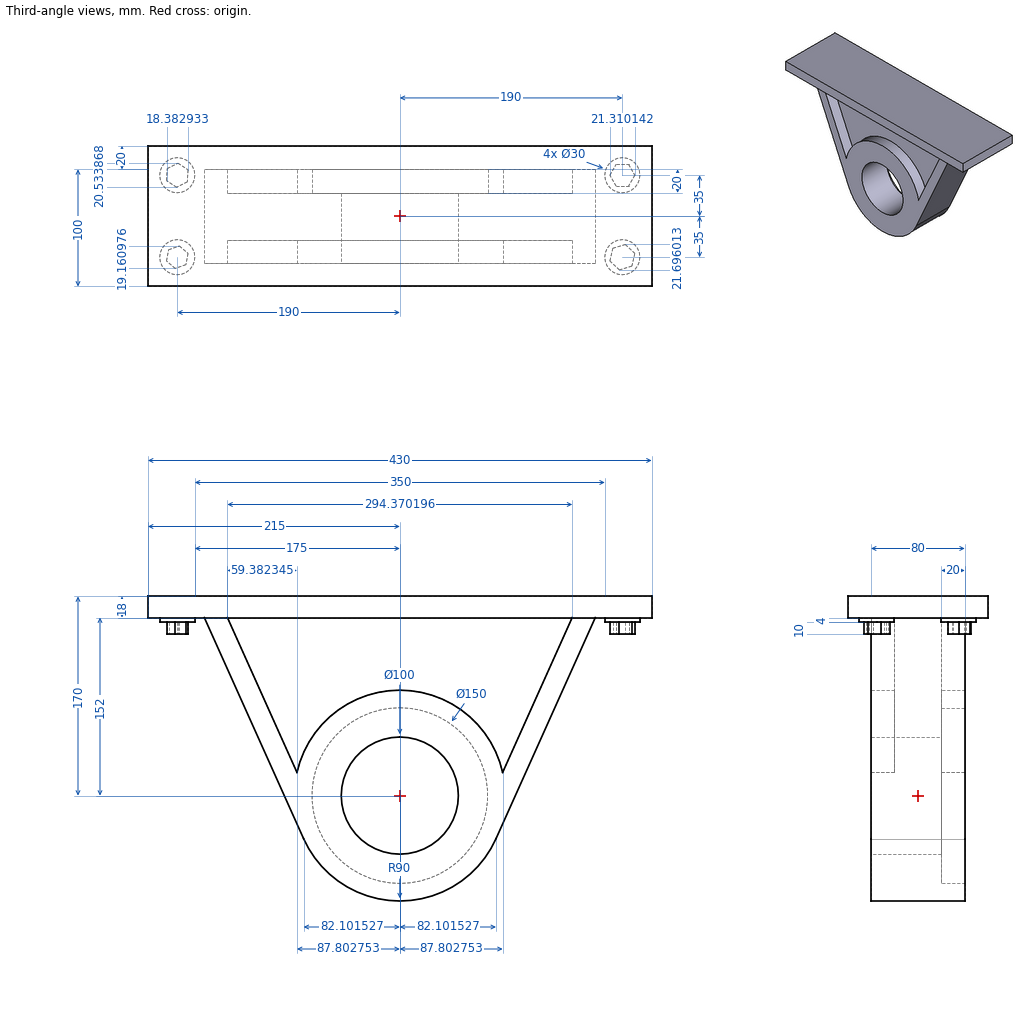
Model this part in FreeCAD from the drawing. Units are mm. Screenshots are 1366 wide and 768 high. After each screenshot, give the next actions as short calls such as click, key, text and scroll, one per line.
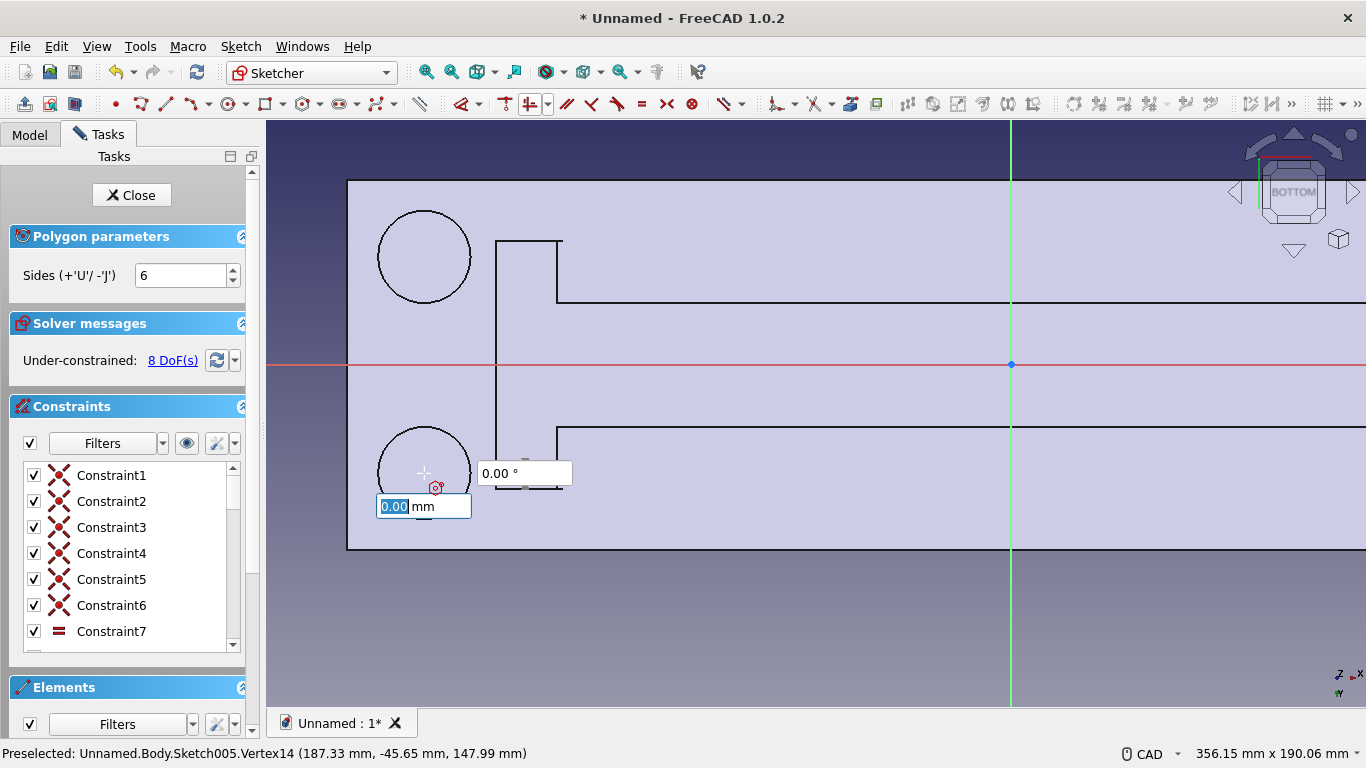
click(426, 505)
right_click(426, 505)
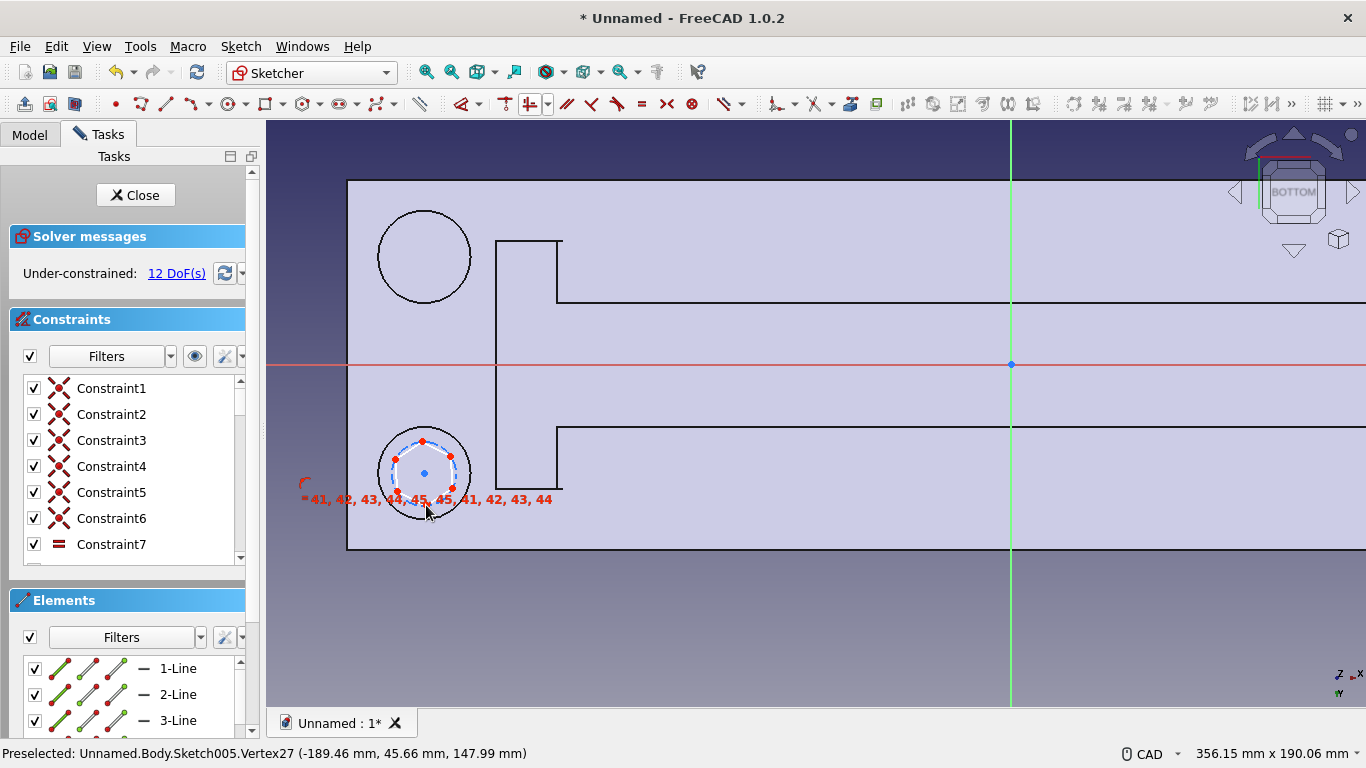
click(302, 104)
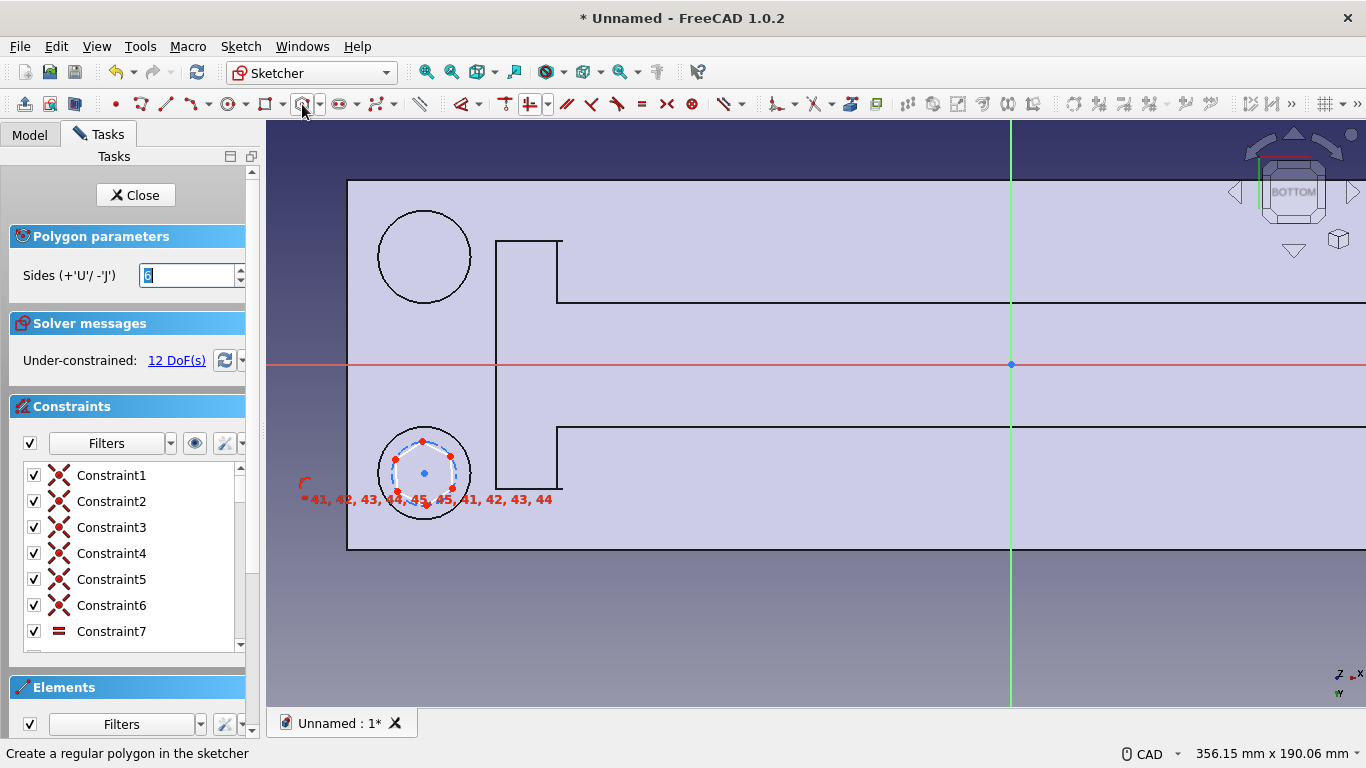
click(424, 257)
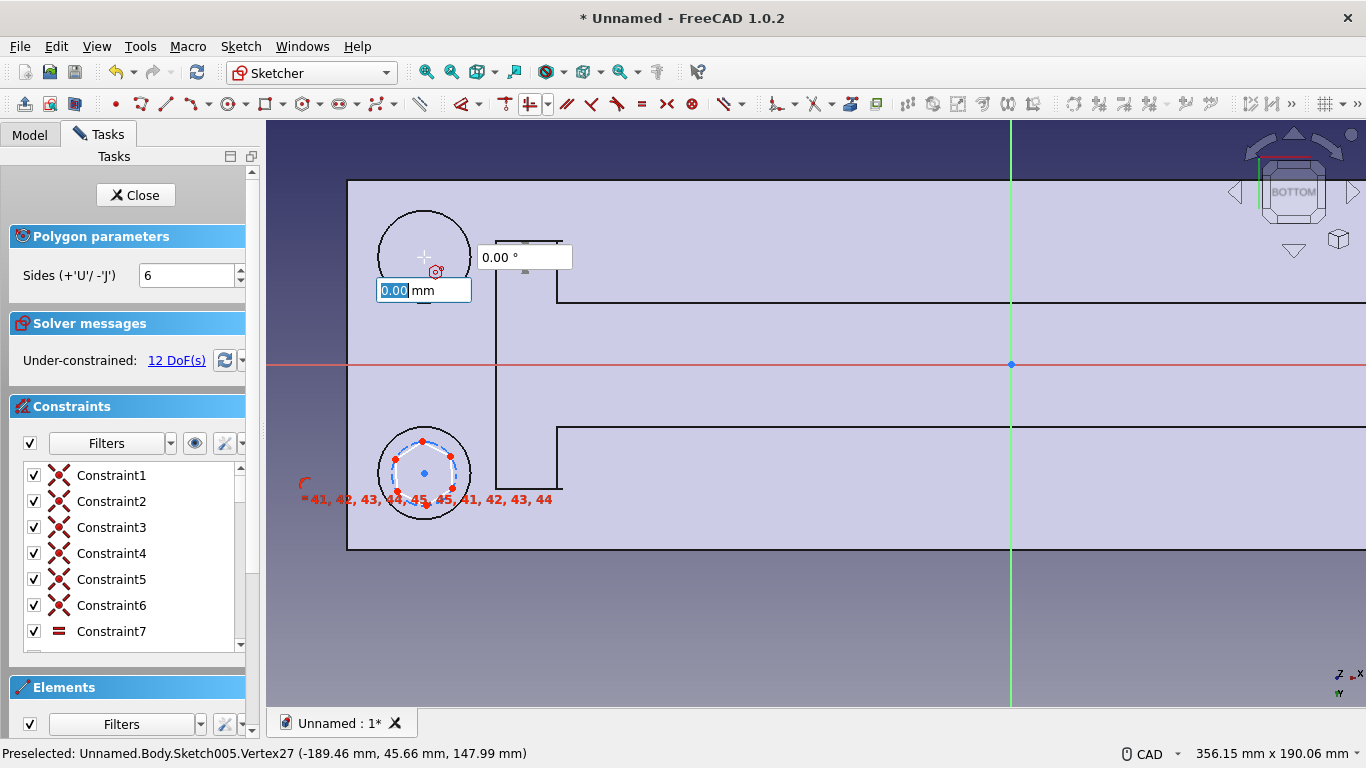
click(419, 227)
right_click(419, 227)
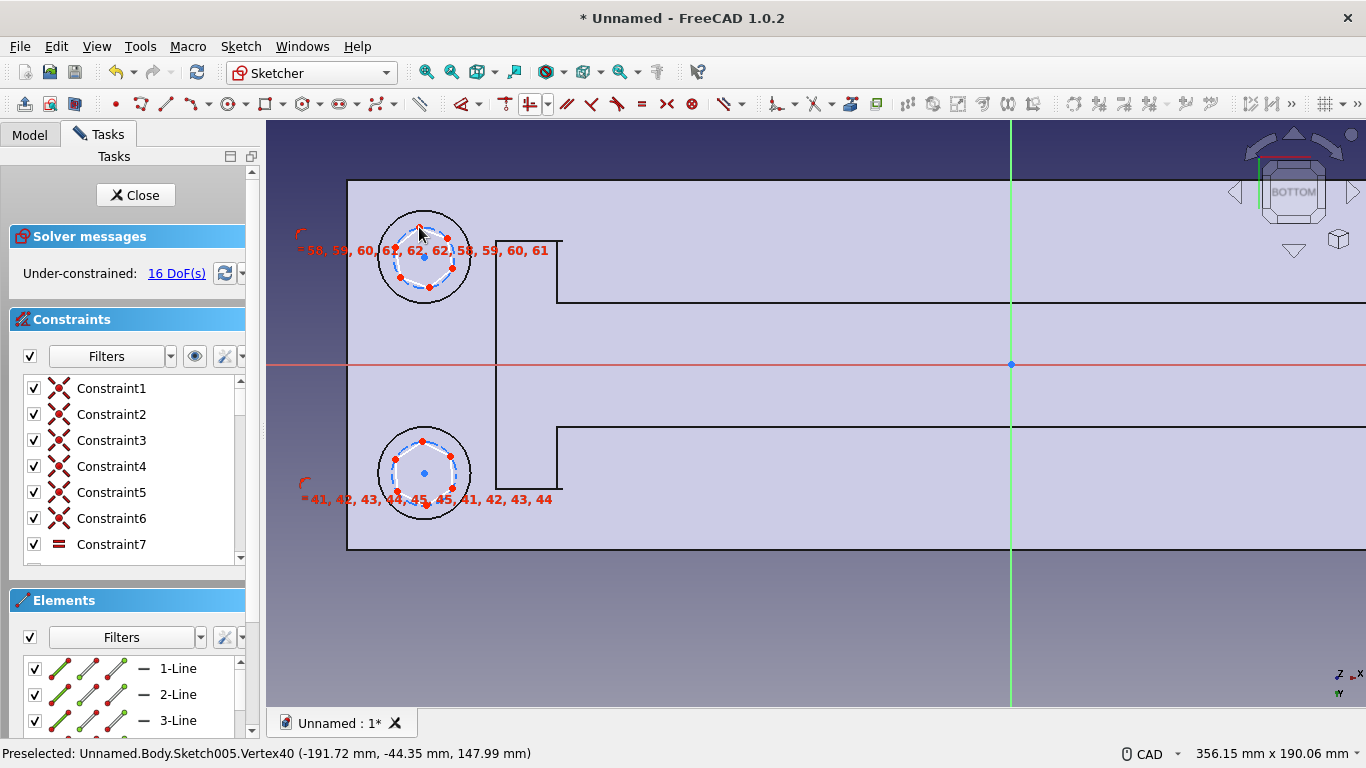
scroll(424, 474, down, 3)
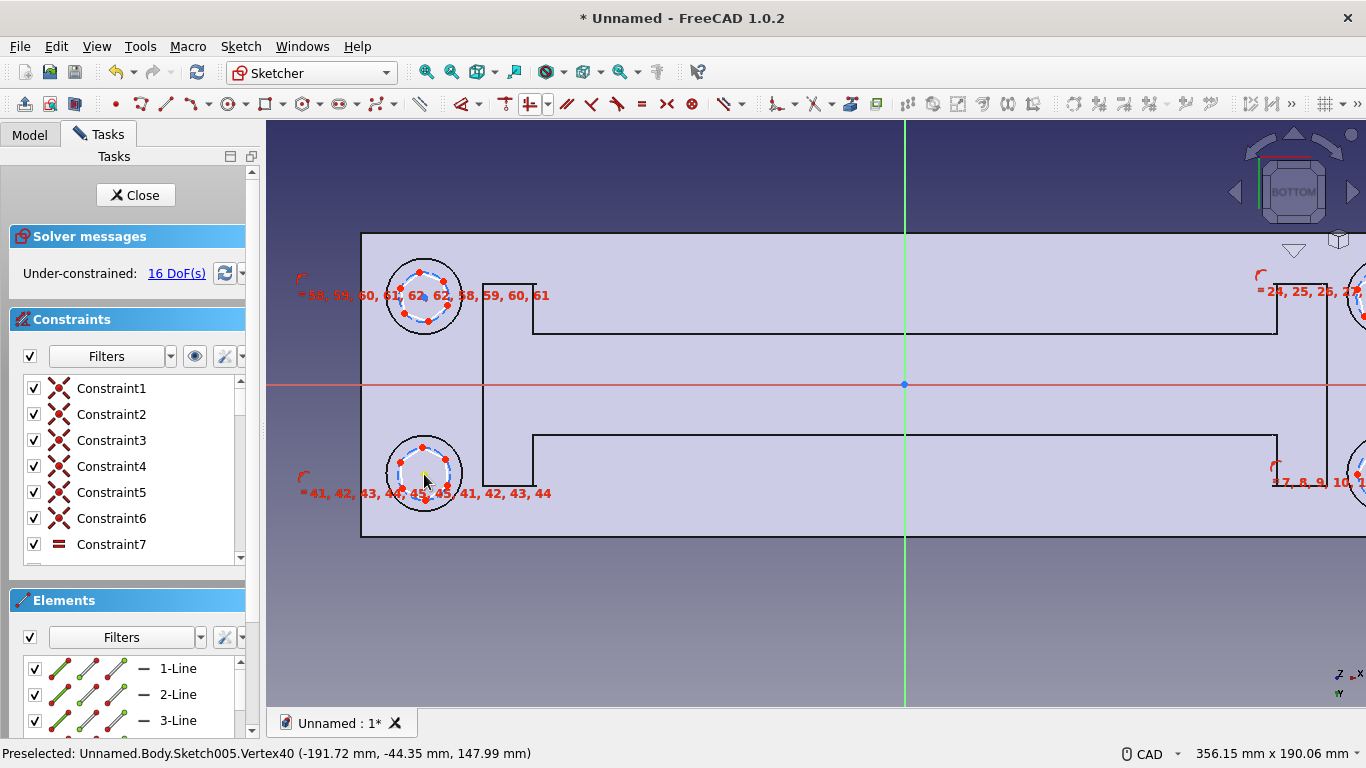
scroll(1068, 490, up, 9)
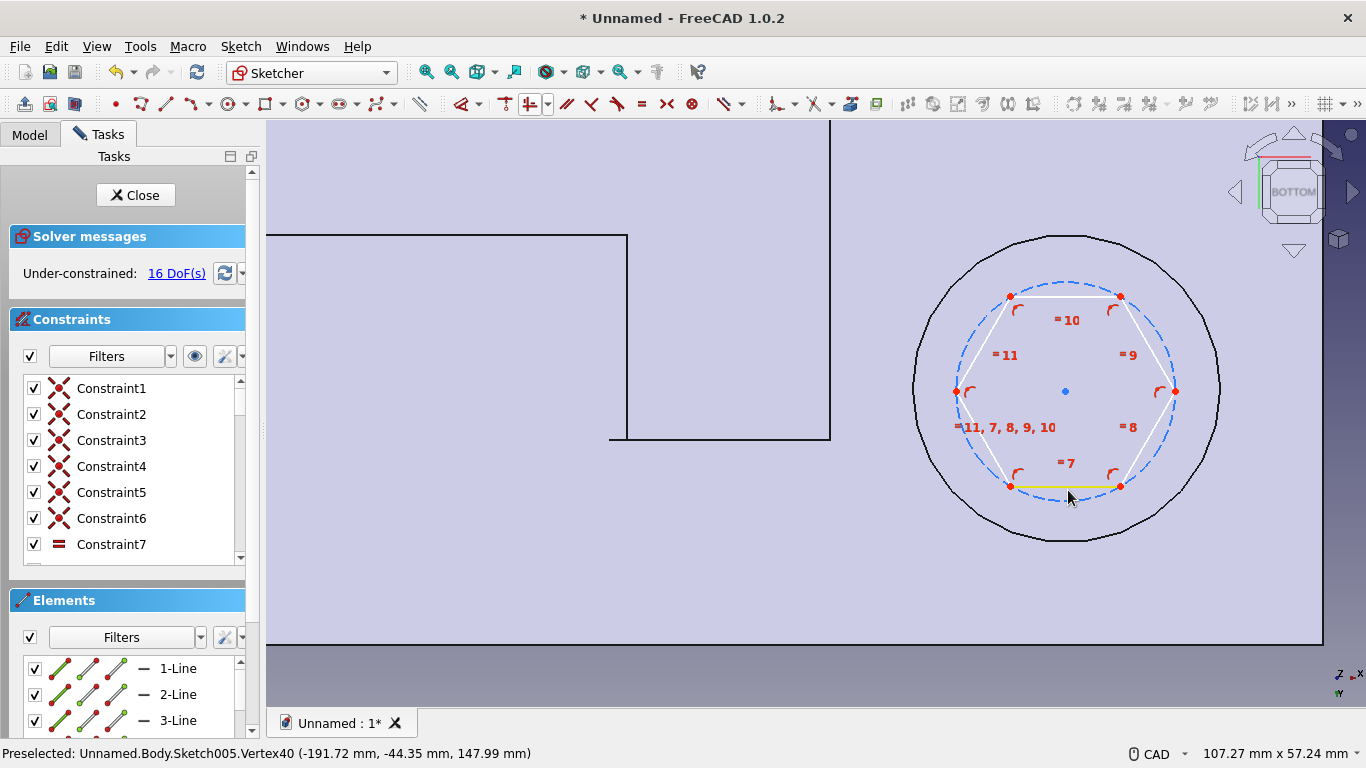
click(1066, 487)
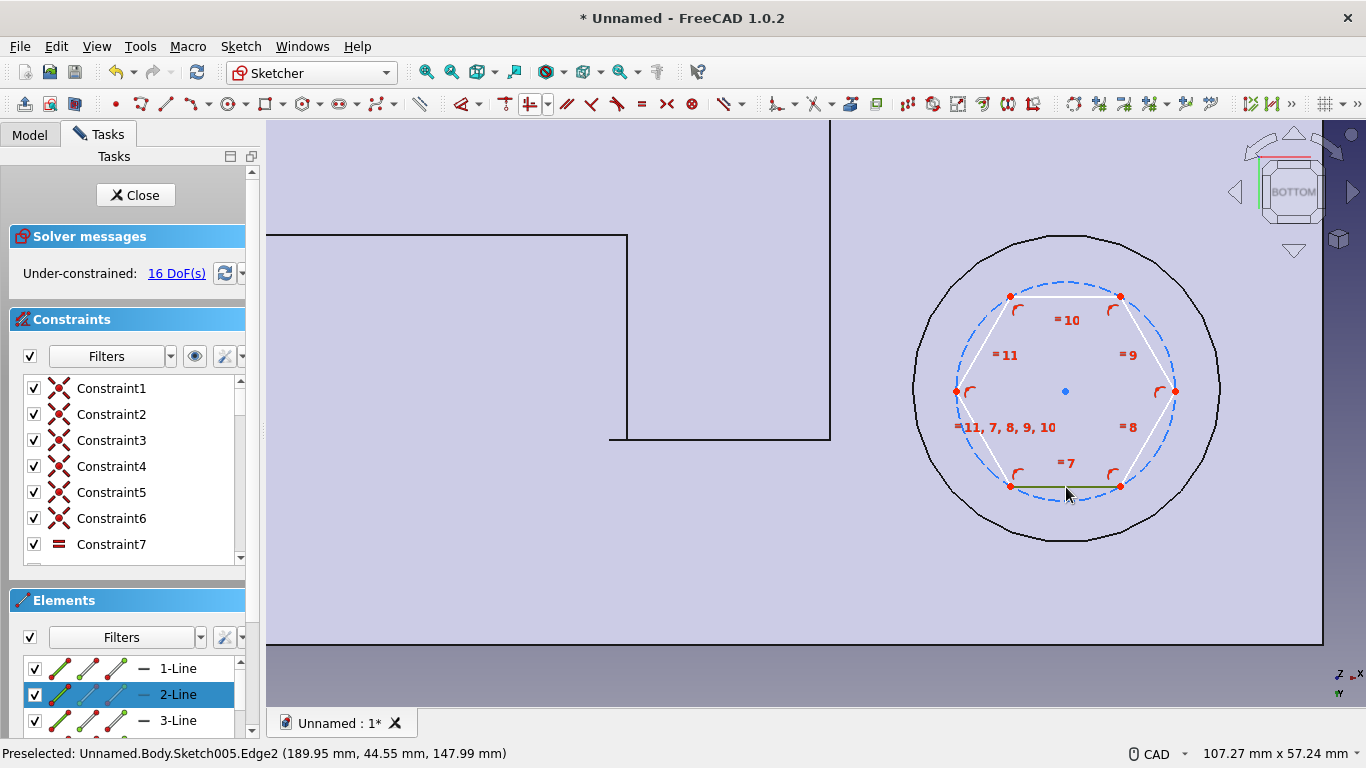
key(h)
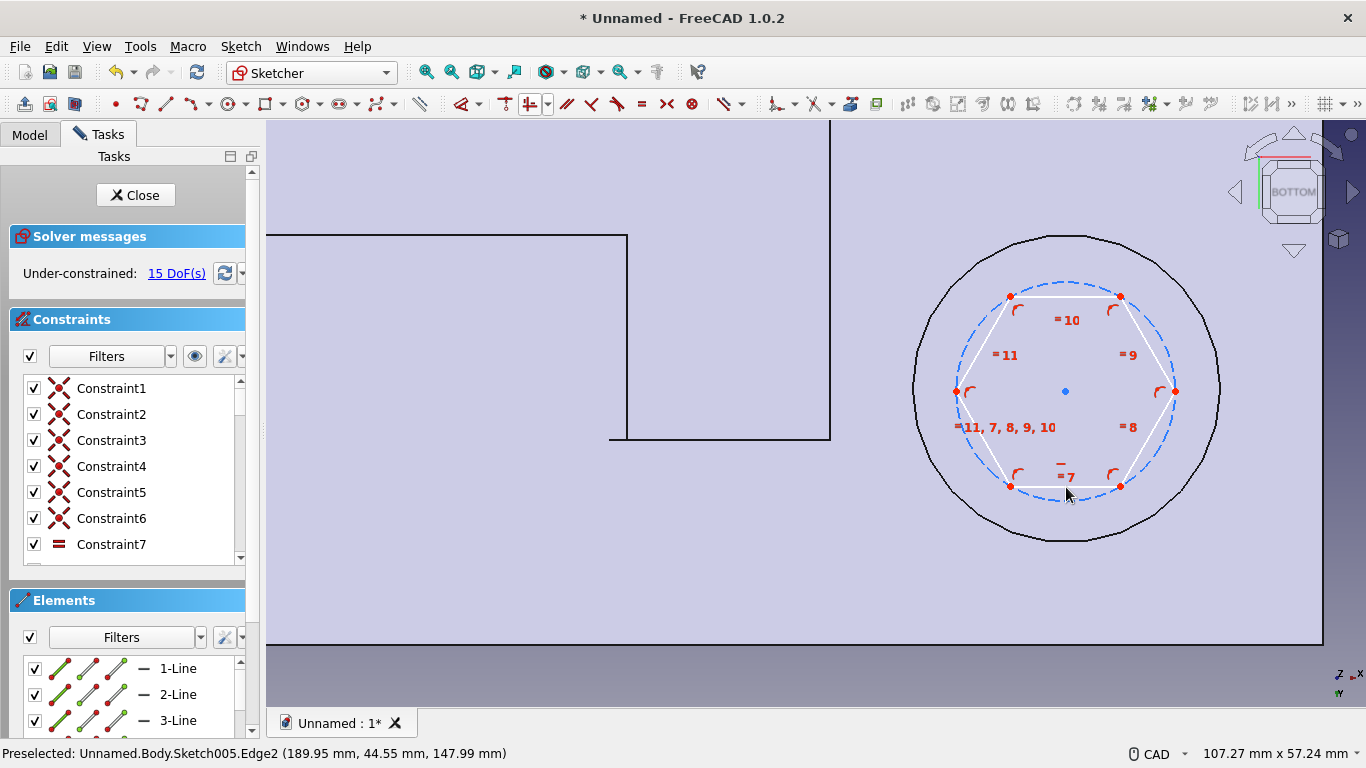
click(460, 104)